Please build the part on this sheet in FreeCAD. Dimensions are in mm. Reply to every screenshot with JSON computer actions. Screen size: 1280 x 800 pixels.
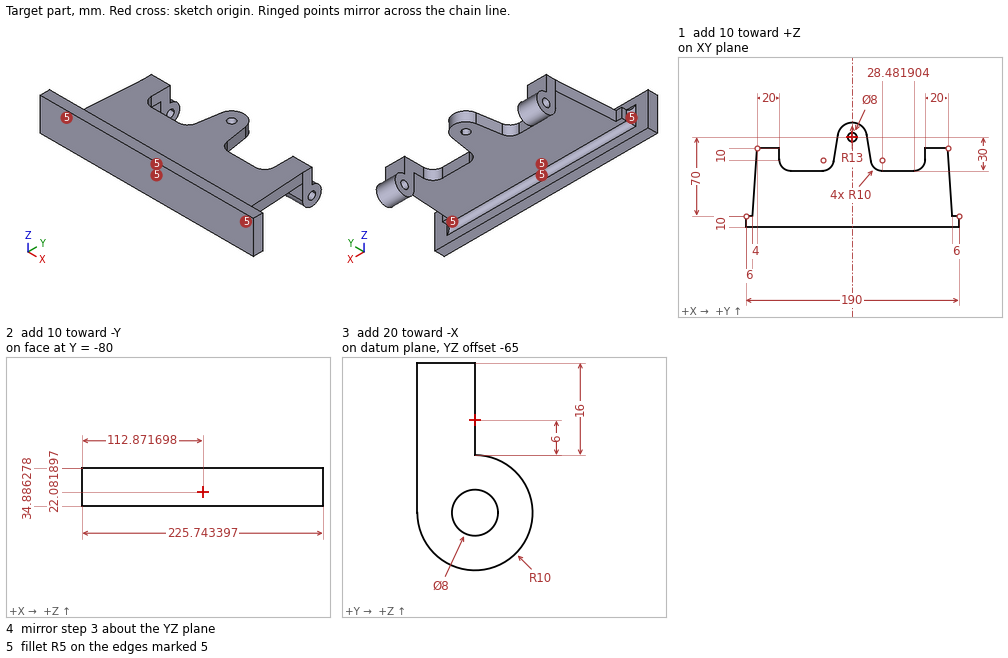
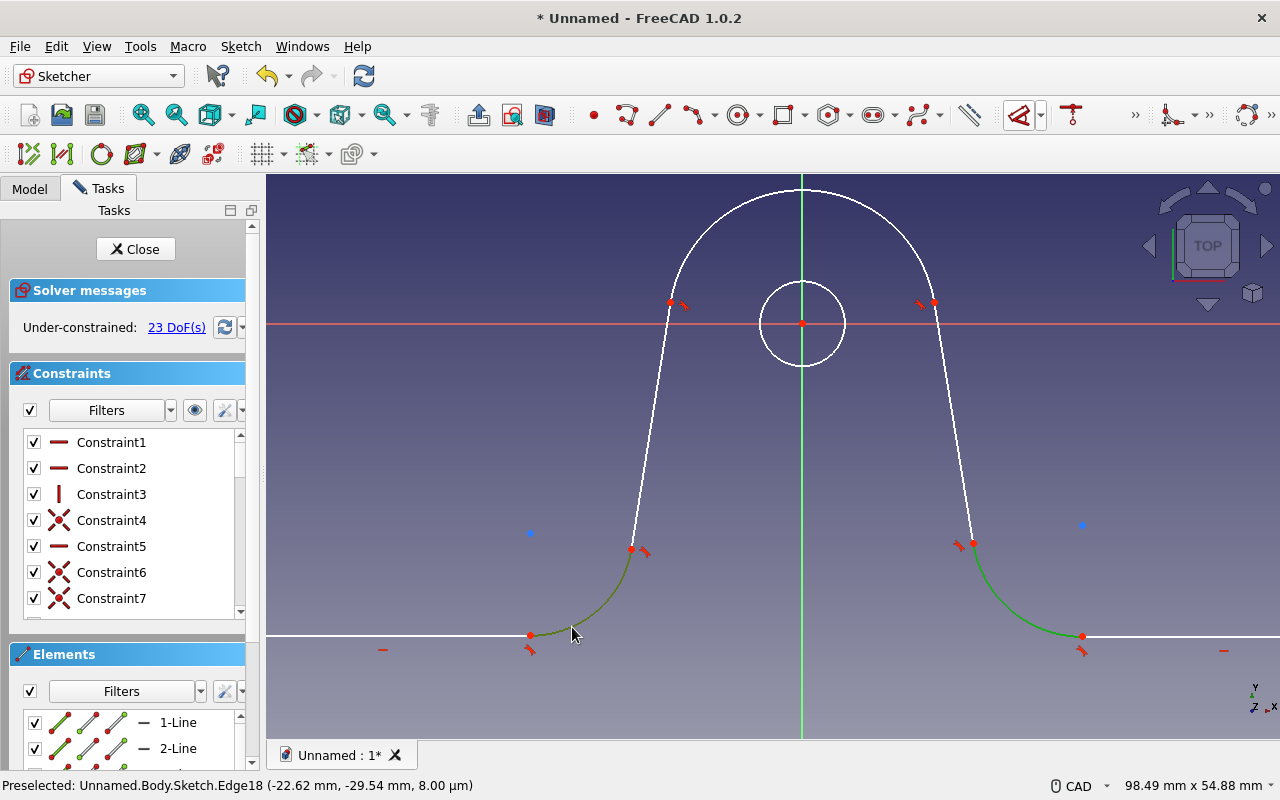
{"action": "scroll", "coordinate": [662, 365], "scroll_direction": "down", "scroll_amount": 6}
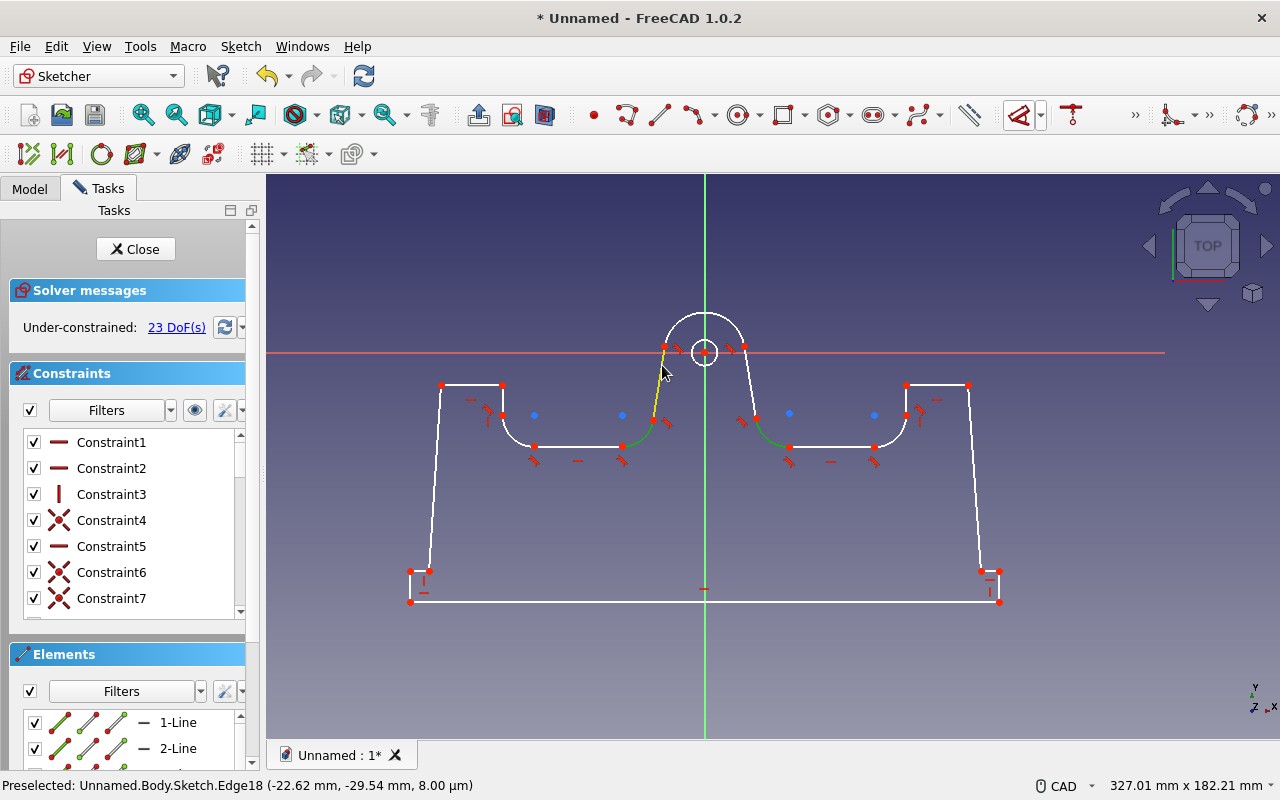
{"action": "left_click", "coordinate": [506, 430]}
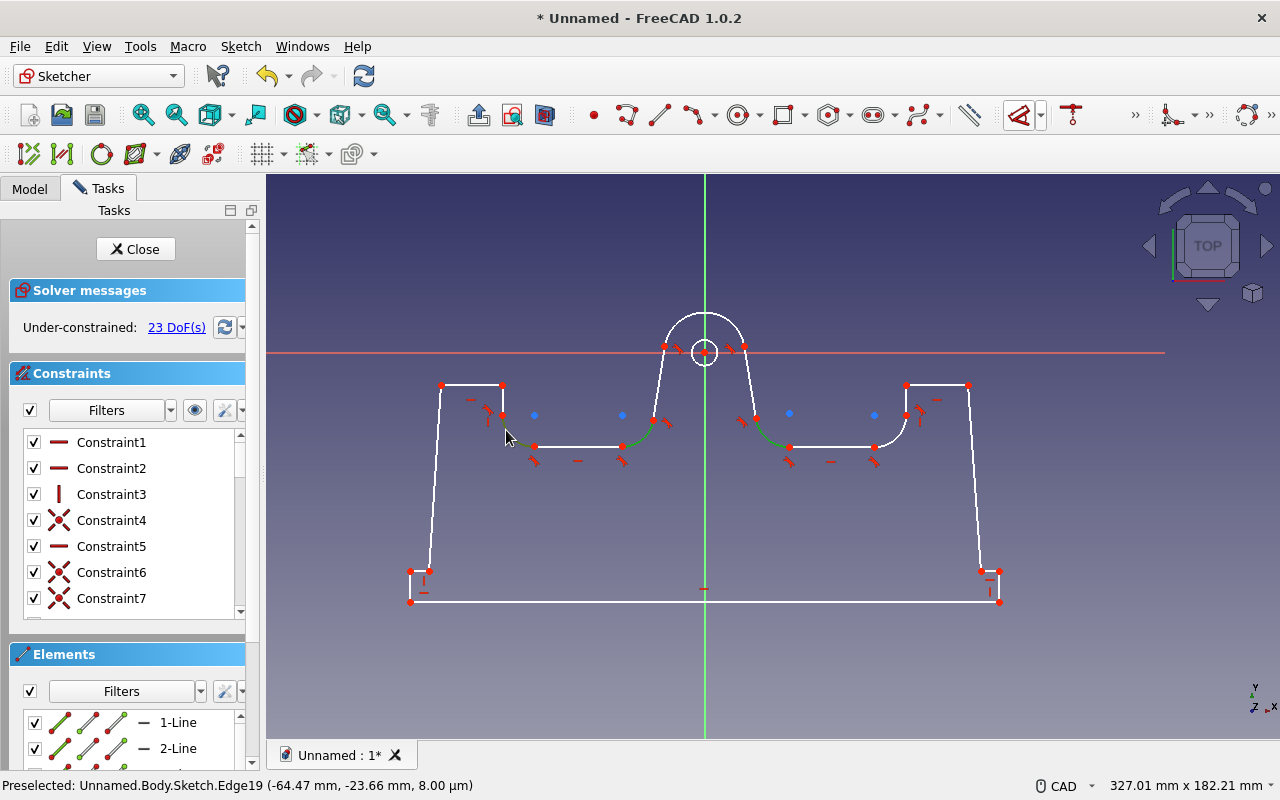
{"action": "left_click", "coordinate": [889, 444]}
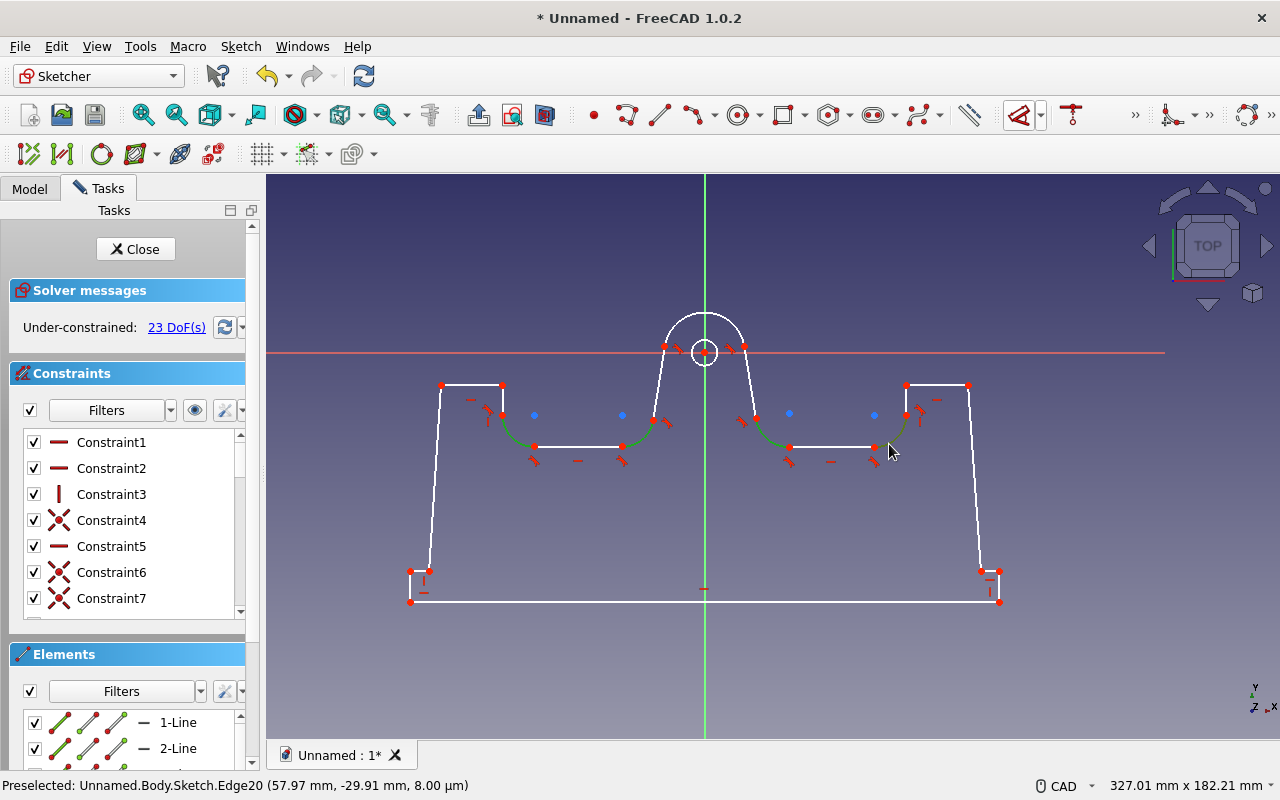
{"action": "key", "text": "e"}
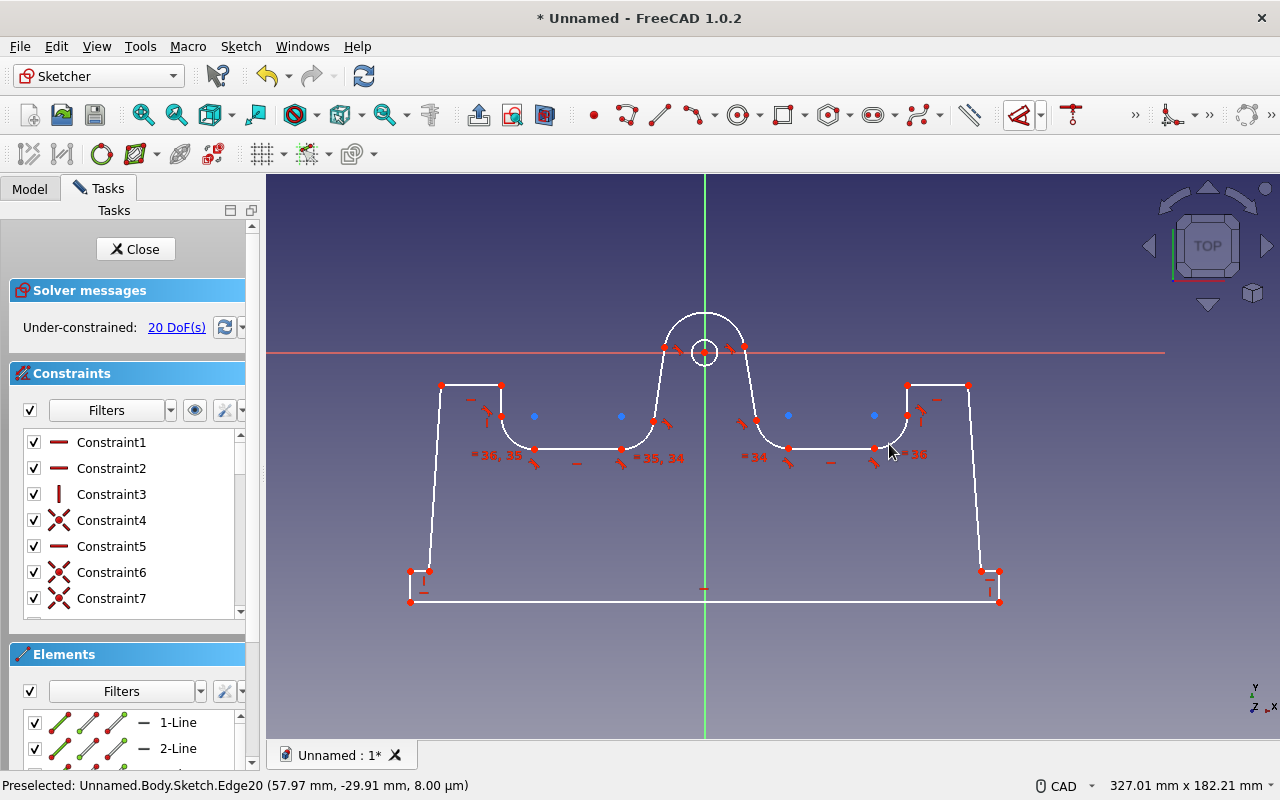
{"action": "left_click", "coordinate": [789, 416]}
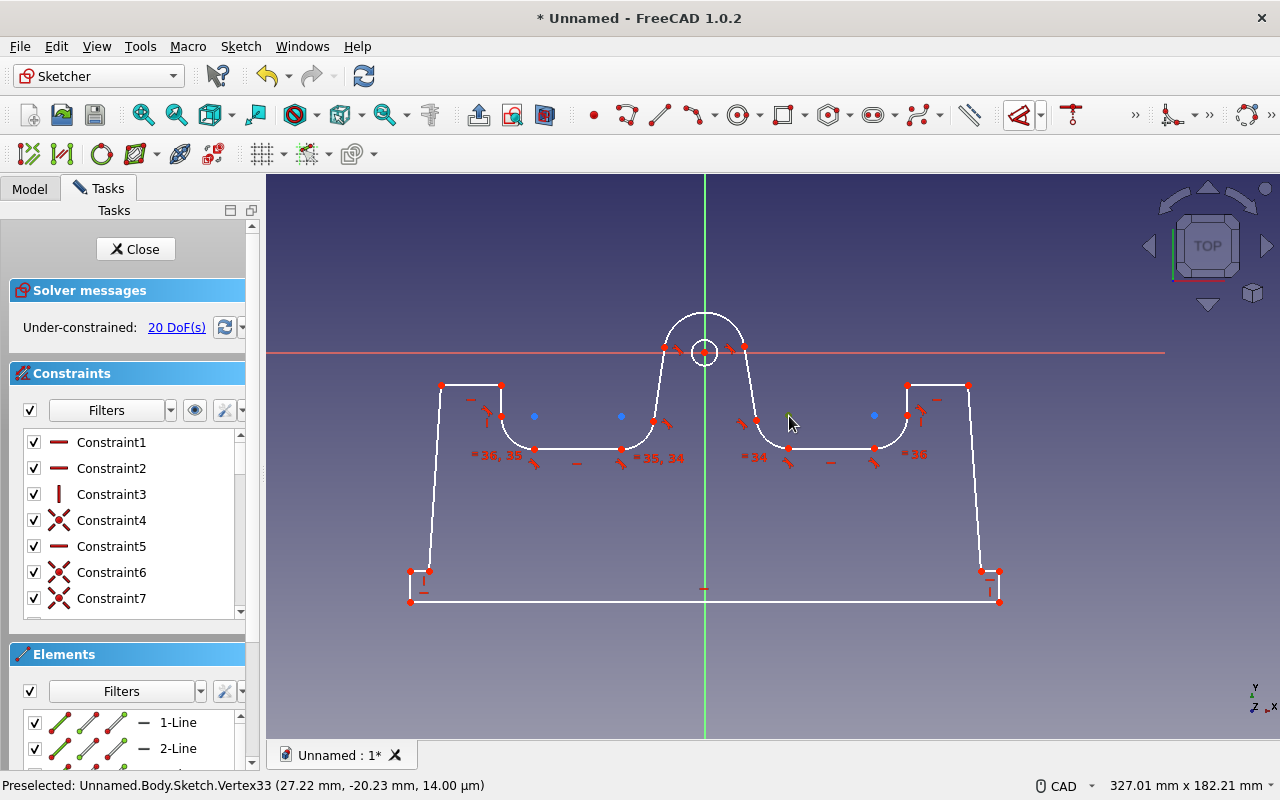
{"action": "left_click", "coordinate": [621, 416]}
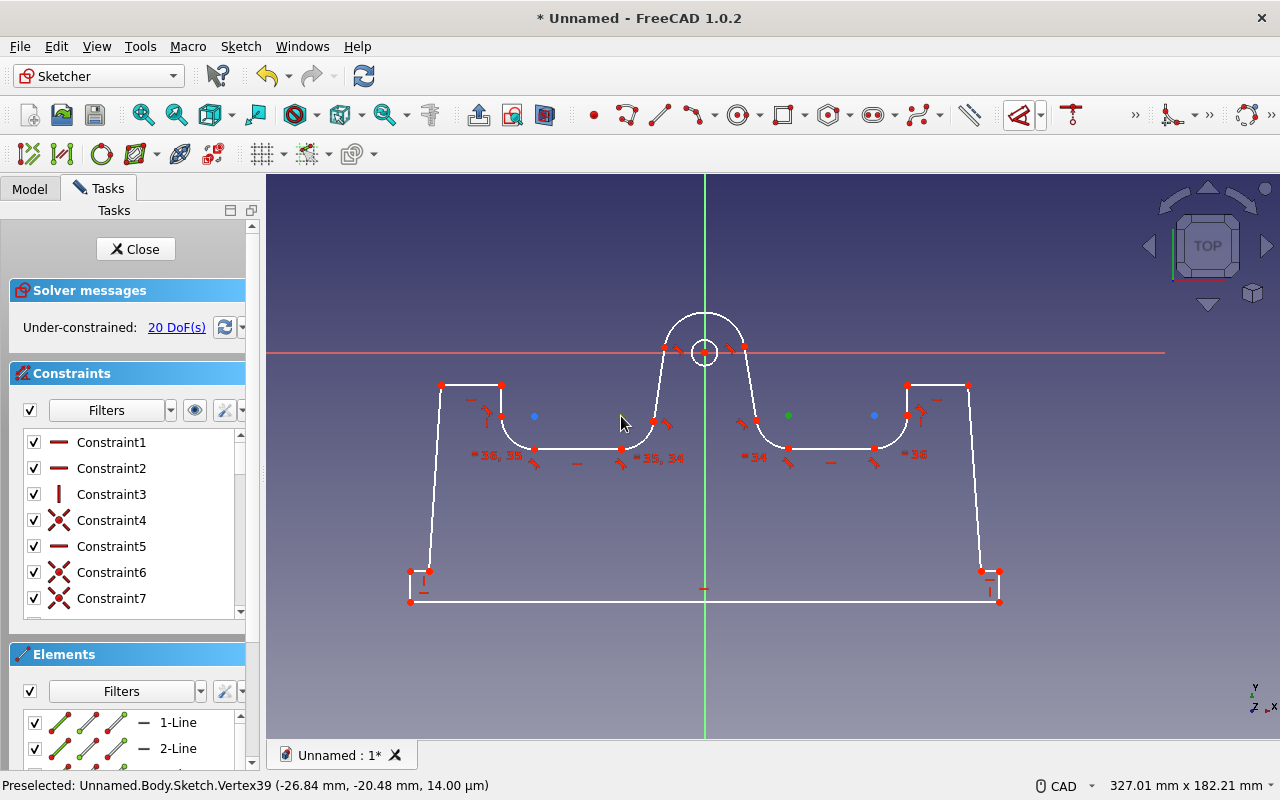
{"action": "left_click", "coordinate": [705, 675]}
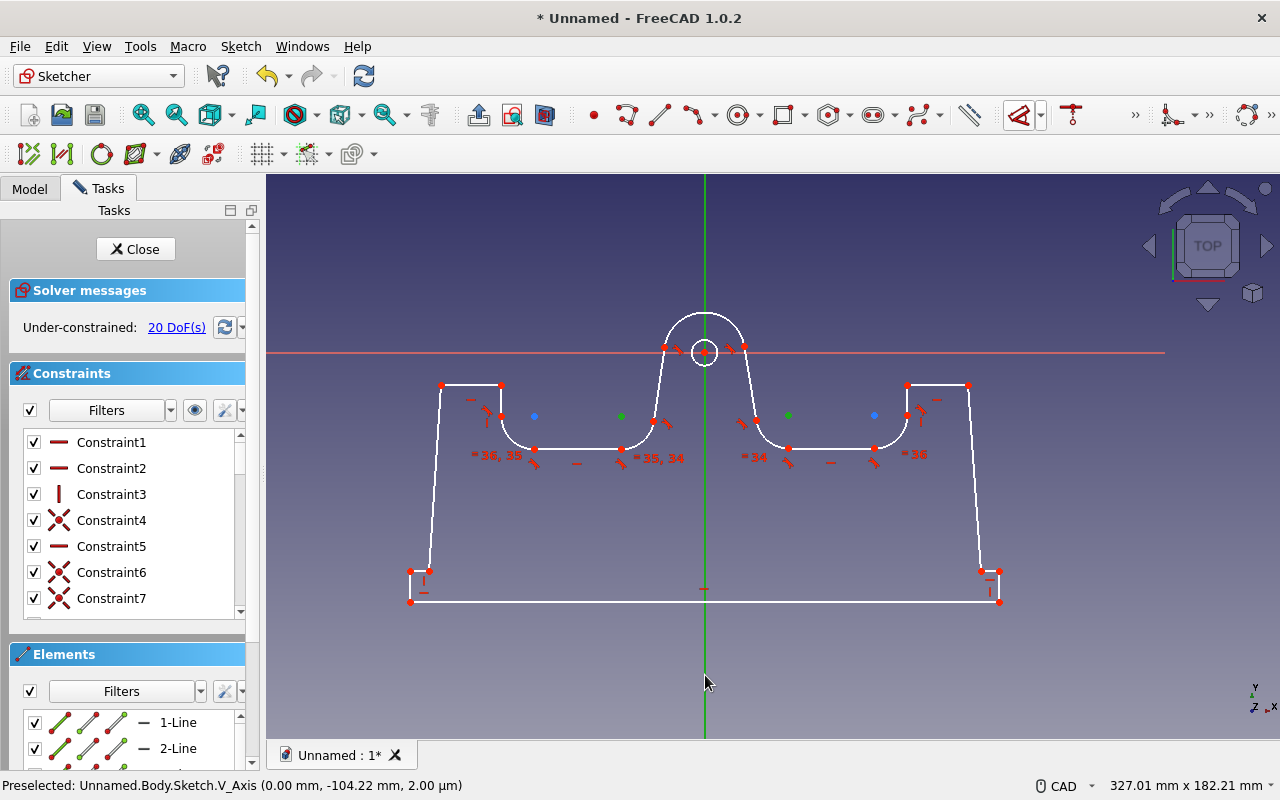
{"action": "key", "text": "s"}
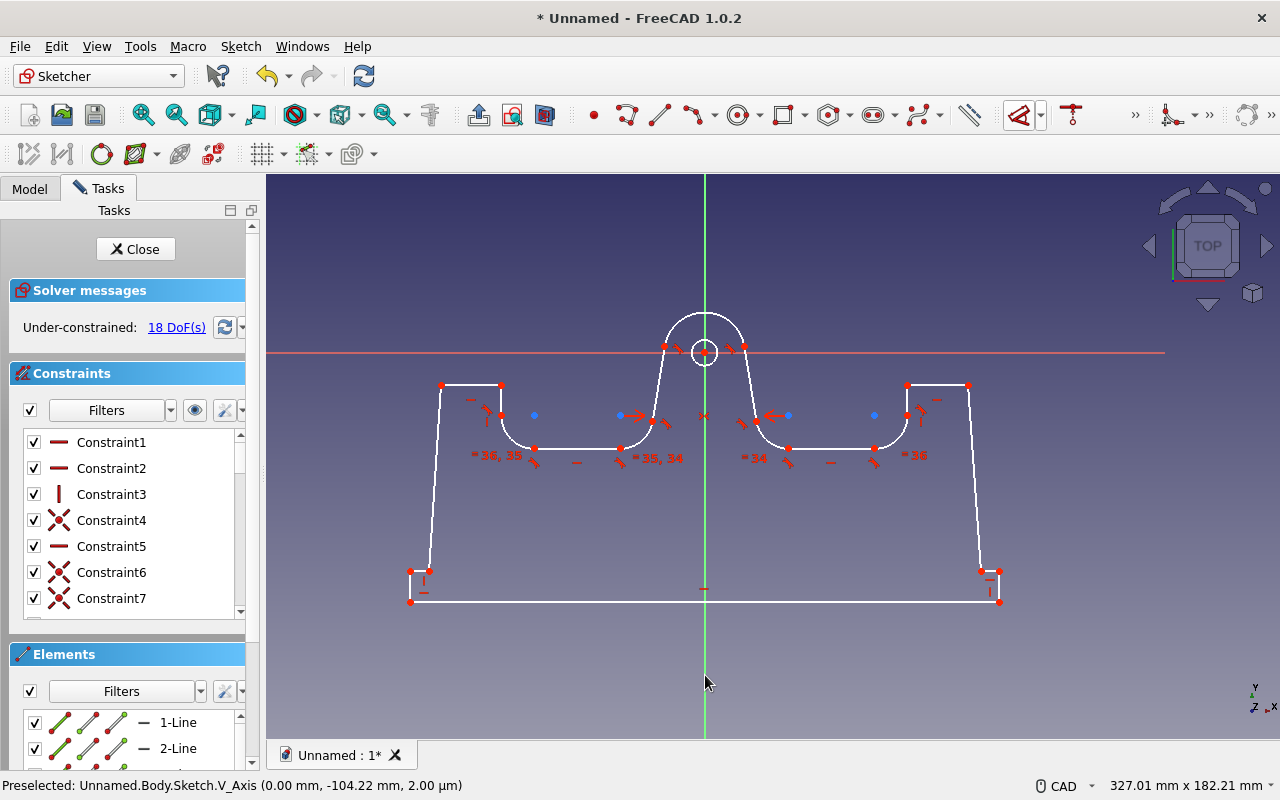
{"action": "left_click", "coordinate": [410, 571]}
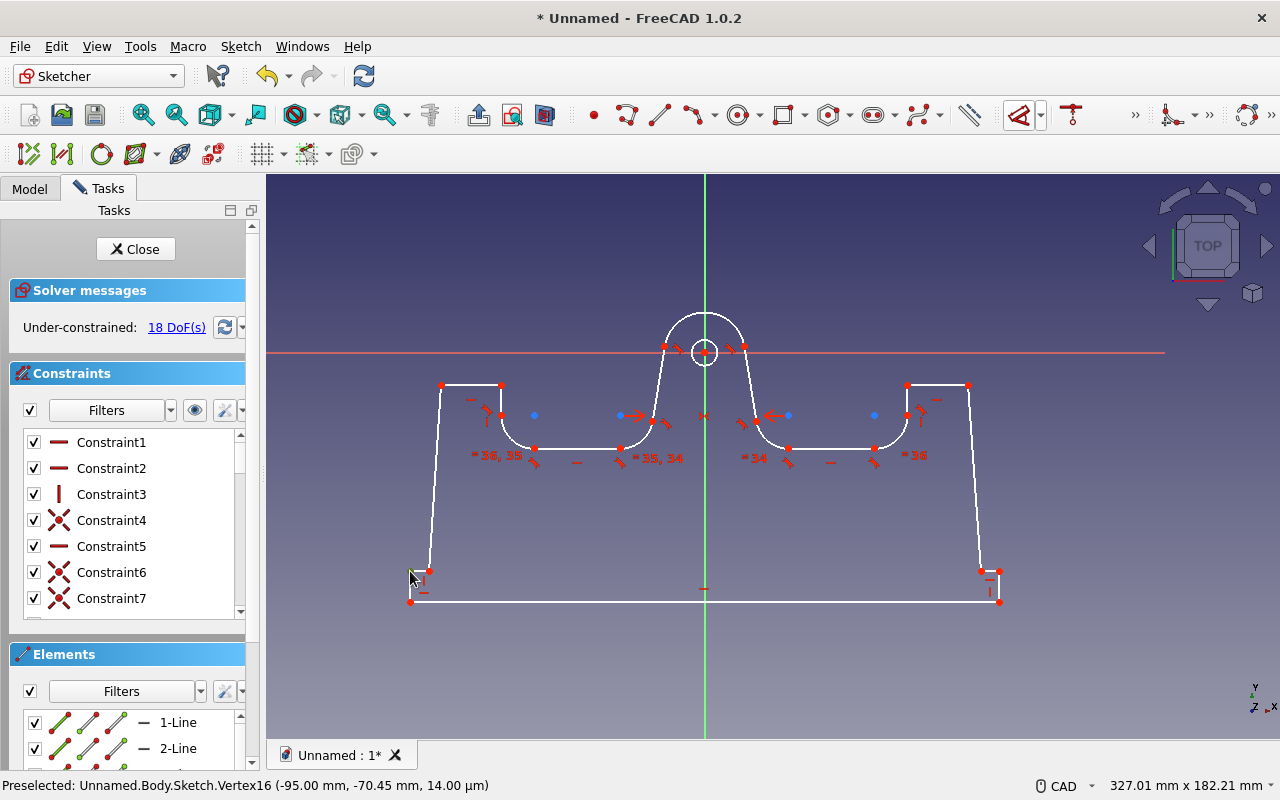
{"action": "left_click", "coordinate": [999, 571]}